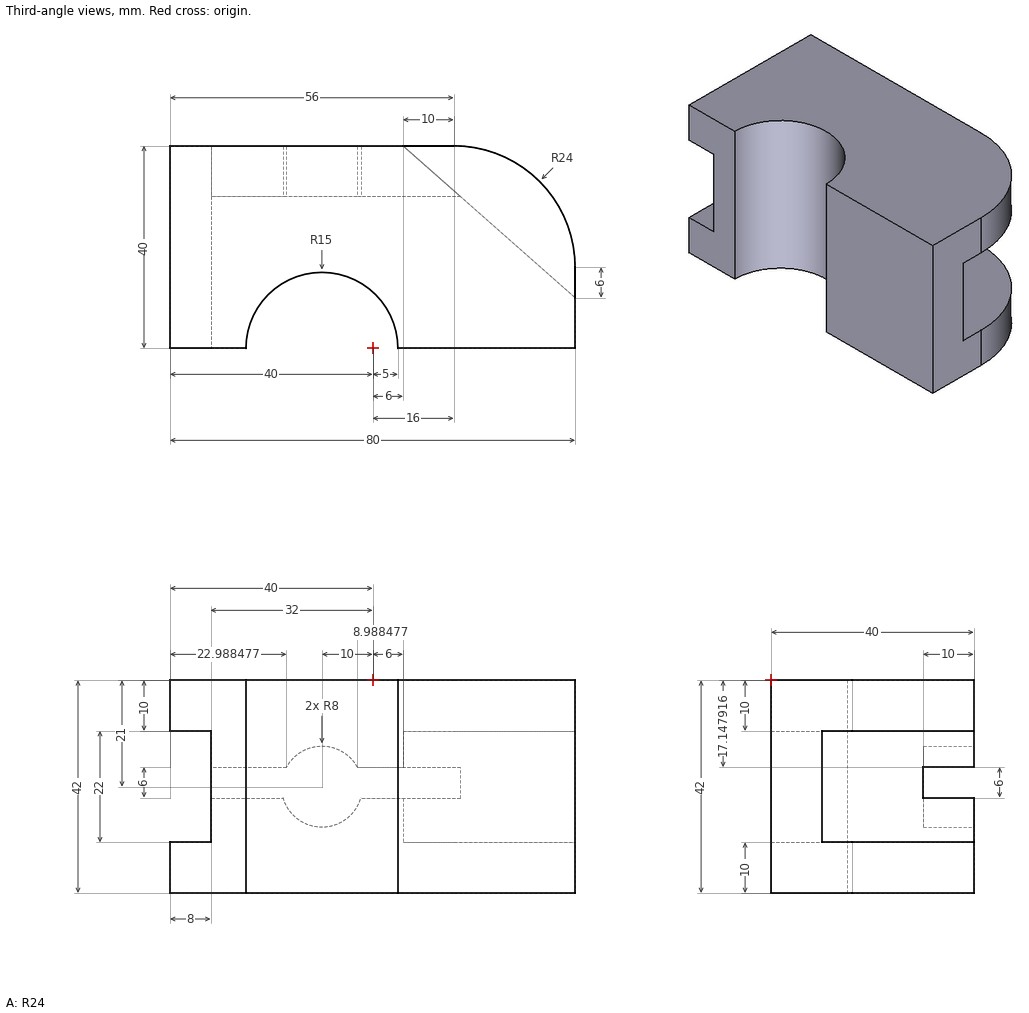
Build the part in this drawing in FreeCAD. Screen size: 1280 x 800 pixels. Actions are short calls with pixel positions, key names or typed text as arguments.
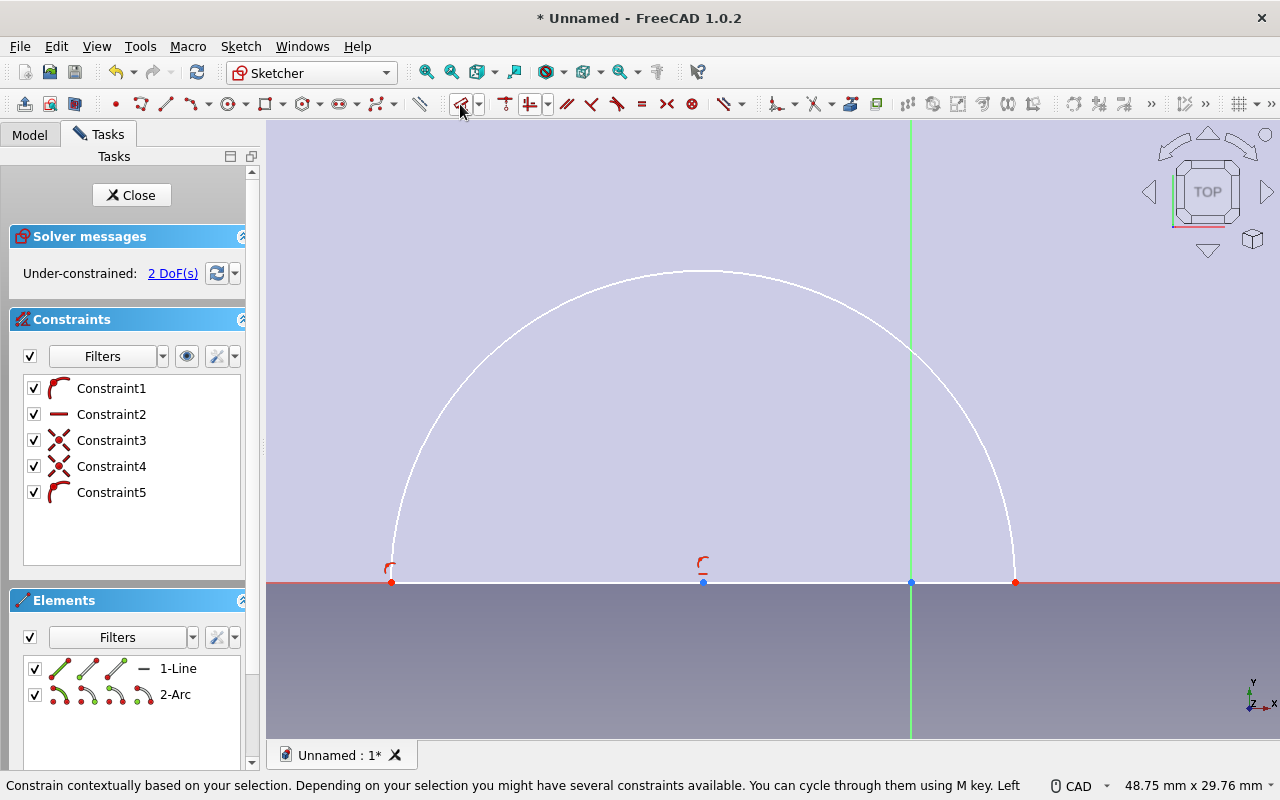
click(886, 330)
click(1014, 435)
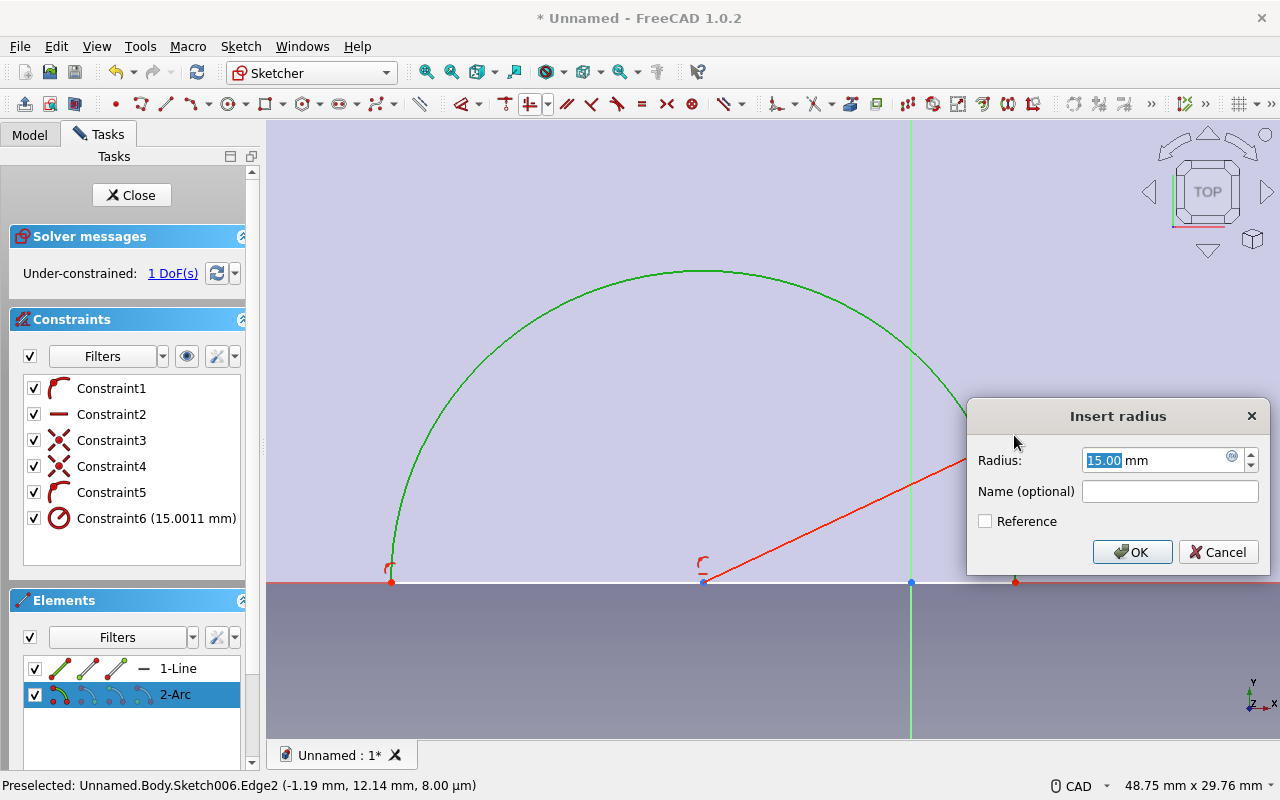
text(15)
key(Return)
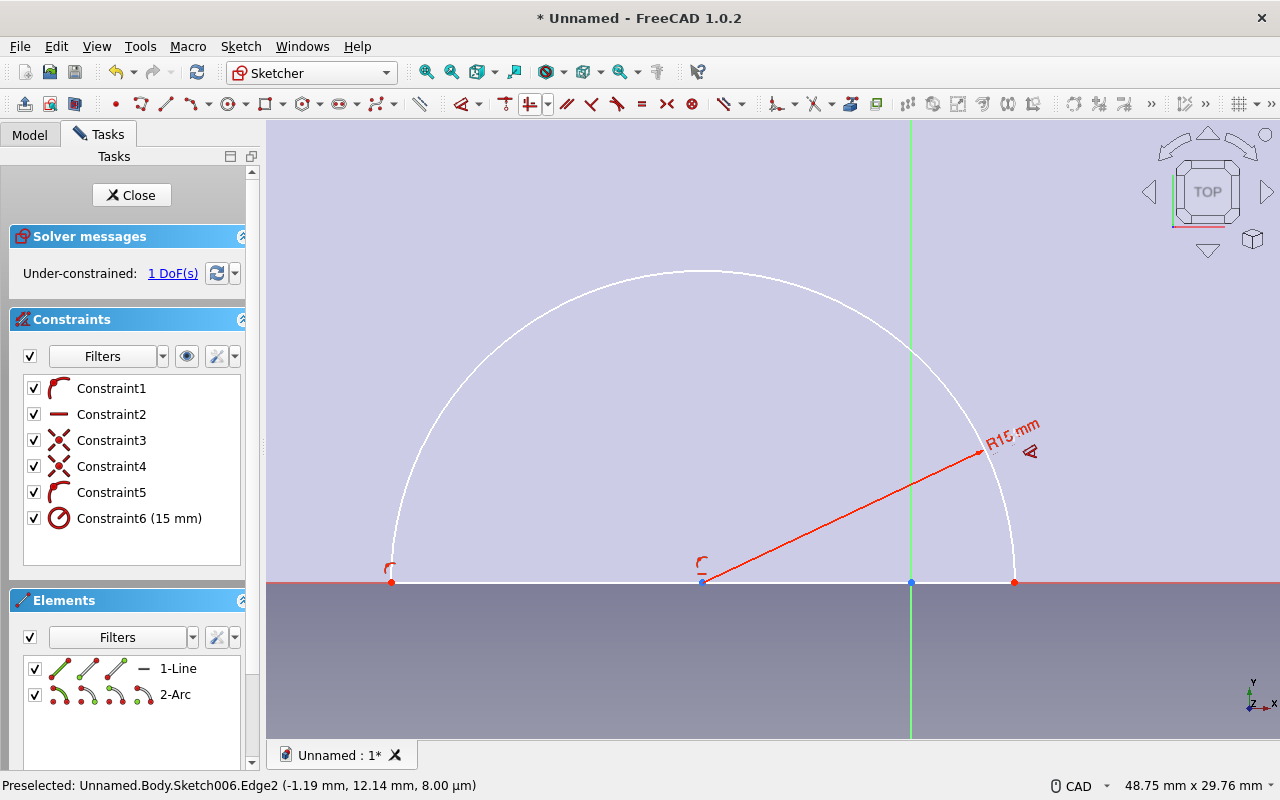
click(1015, 583)
click(963, 617)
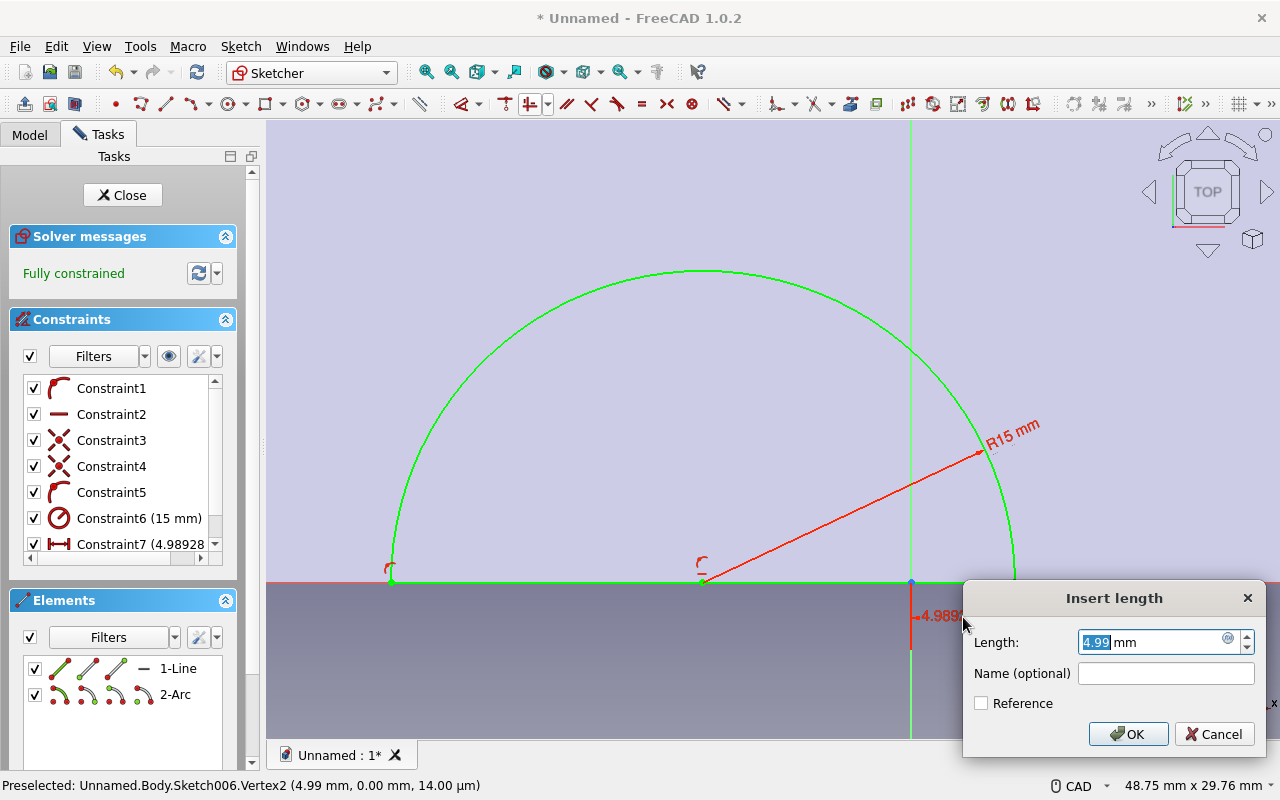
text(5)
key(Return)
key(Escape)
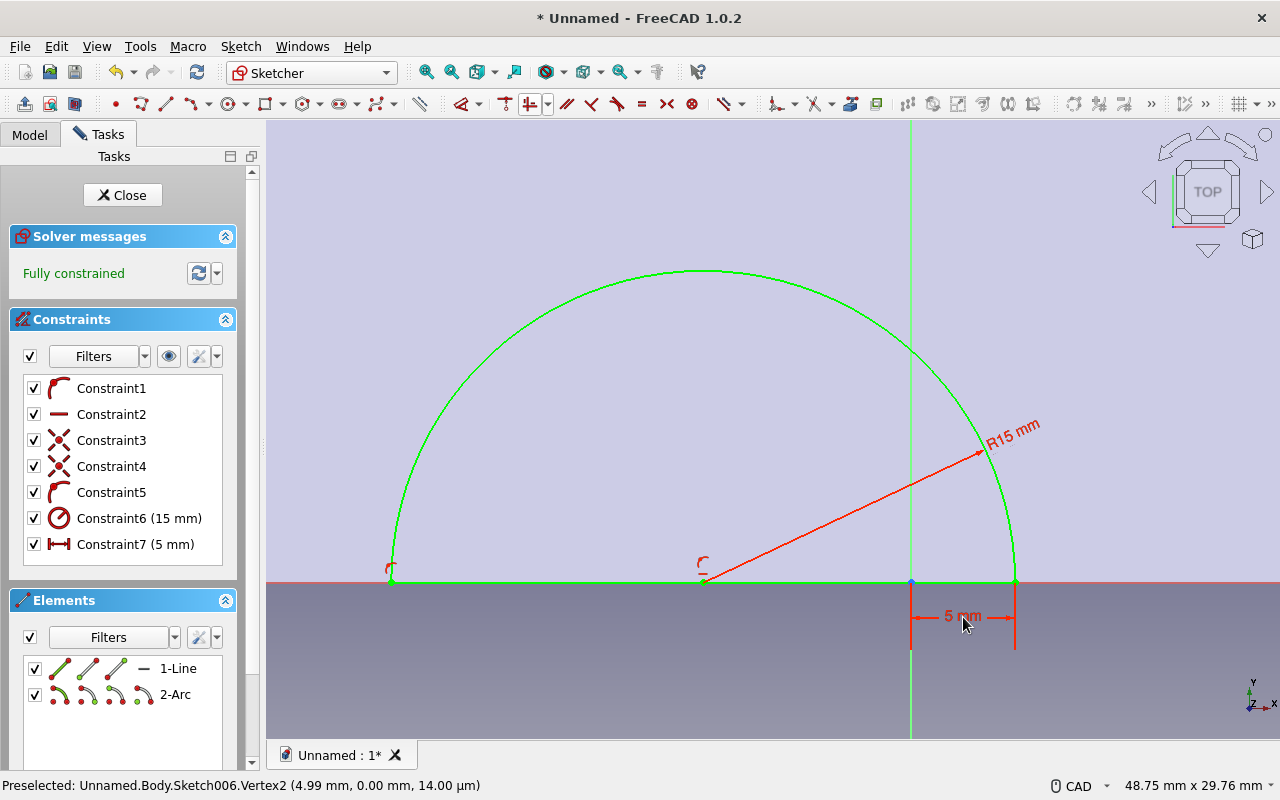
click(123, 195)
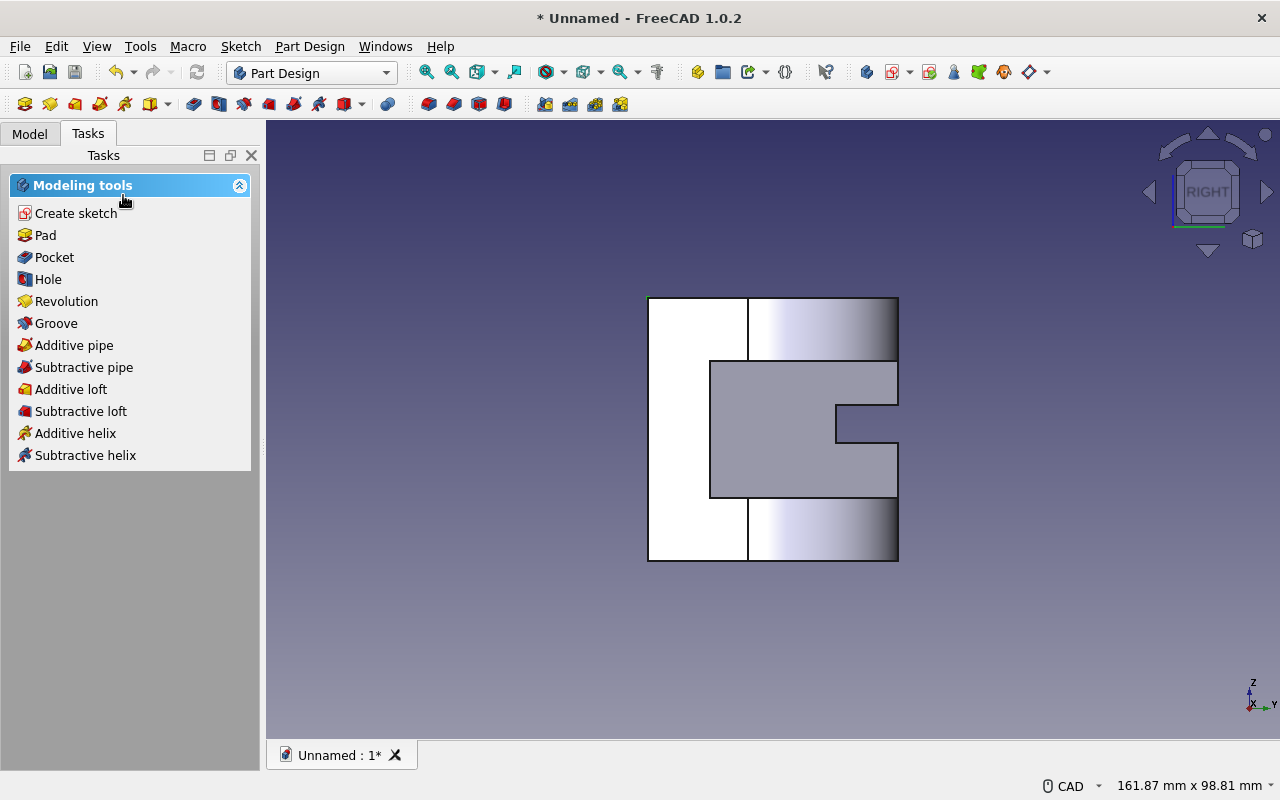
click(194, 104)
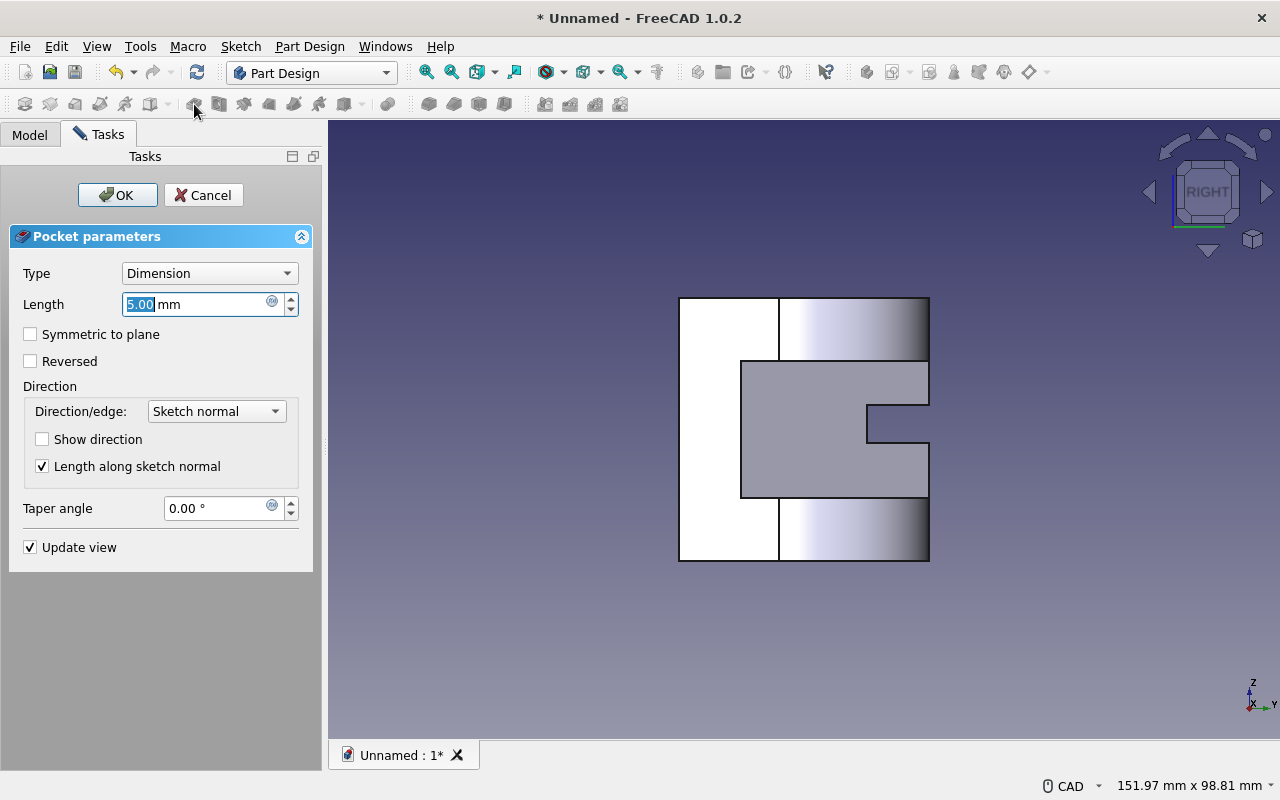
text(42)
key(Tab)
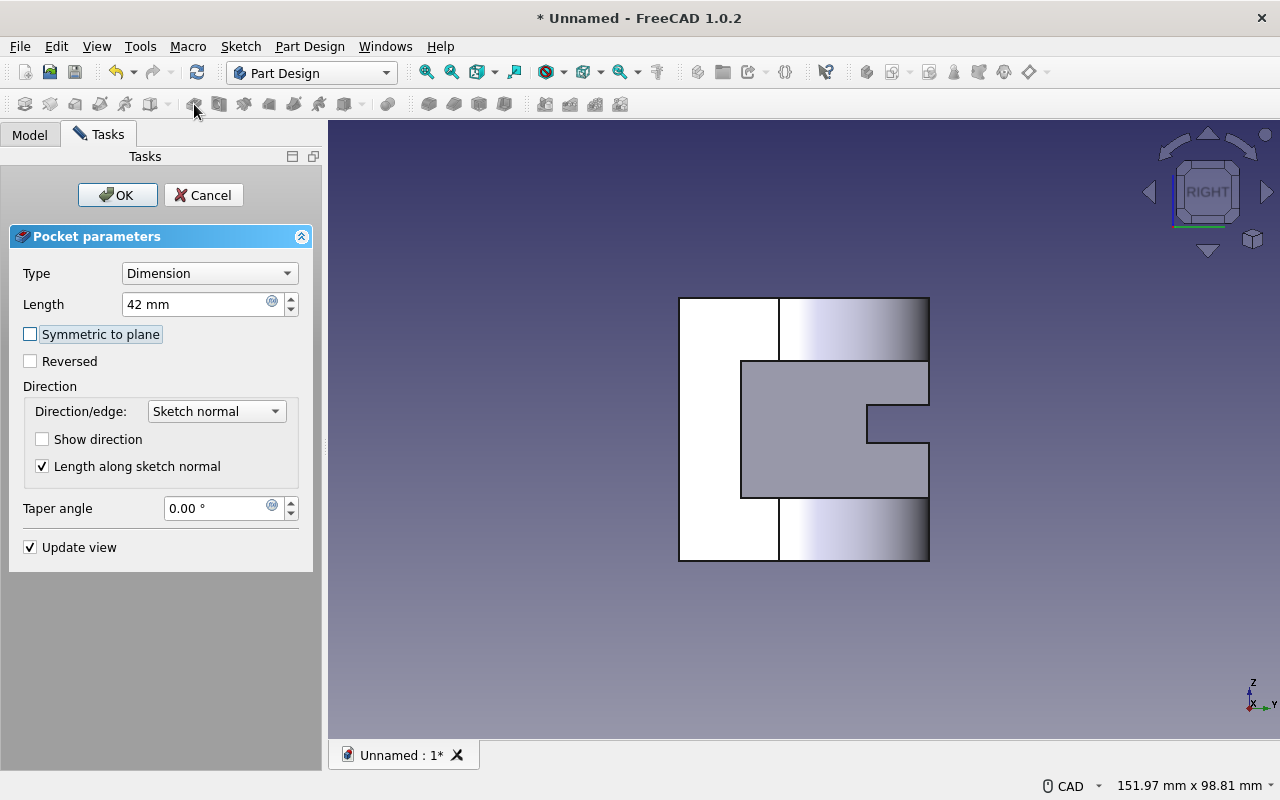
click(118, 195)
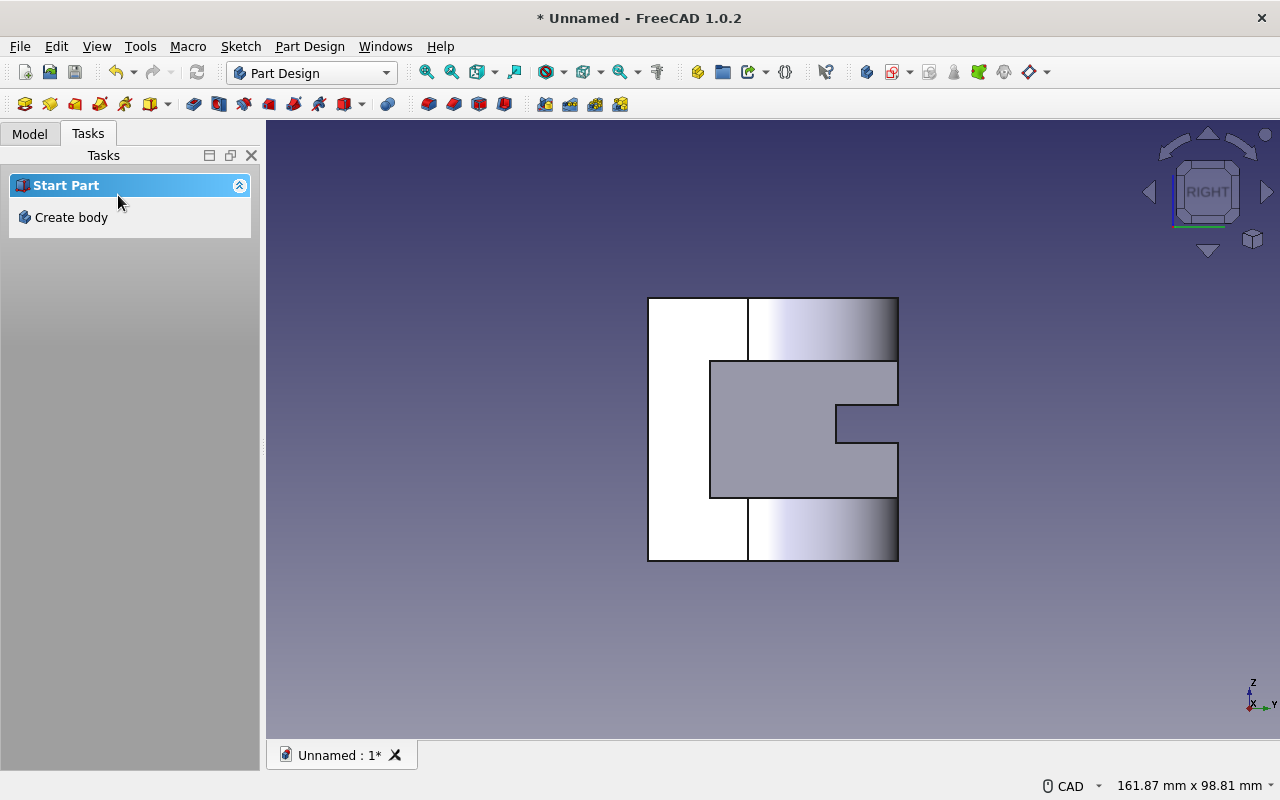
key(v)
key(f)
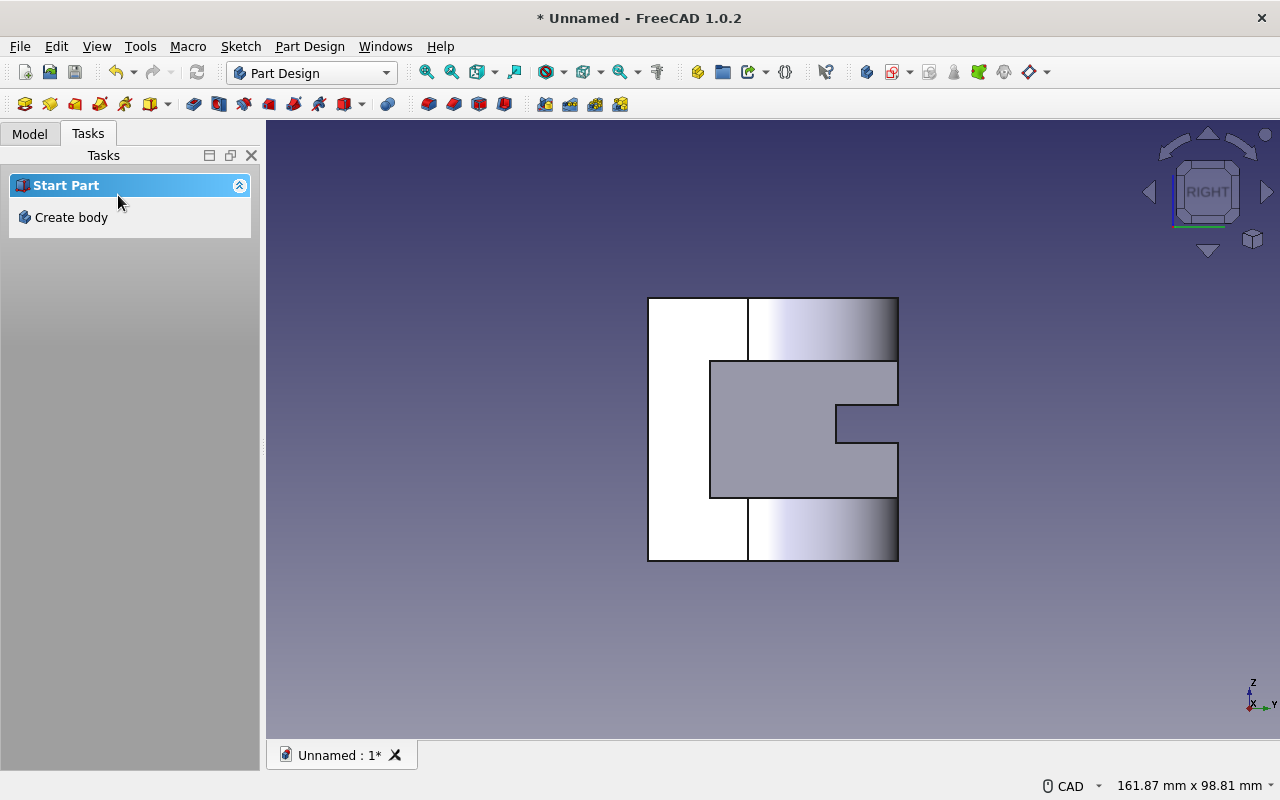
key(4)